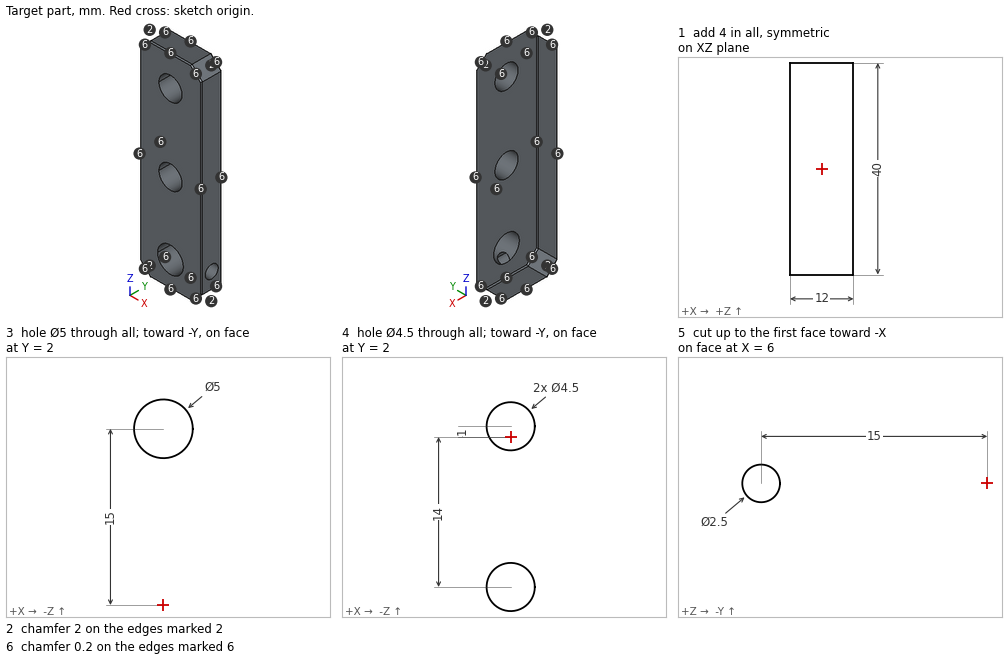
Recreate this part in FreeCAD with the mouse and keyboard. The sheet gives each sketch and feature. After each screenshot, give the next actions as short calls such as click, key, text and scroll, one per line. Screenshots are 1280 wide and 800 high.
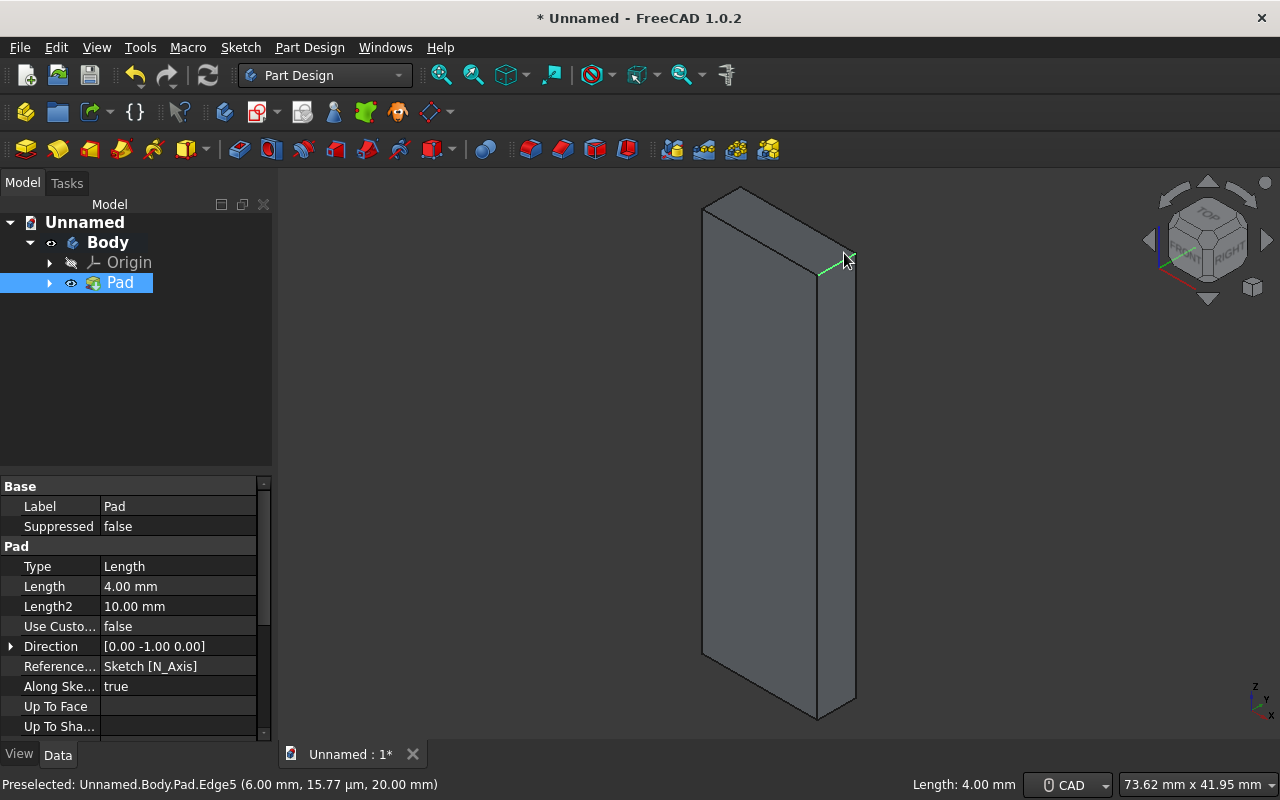
key(2)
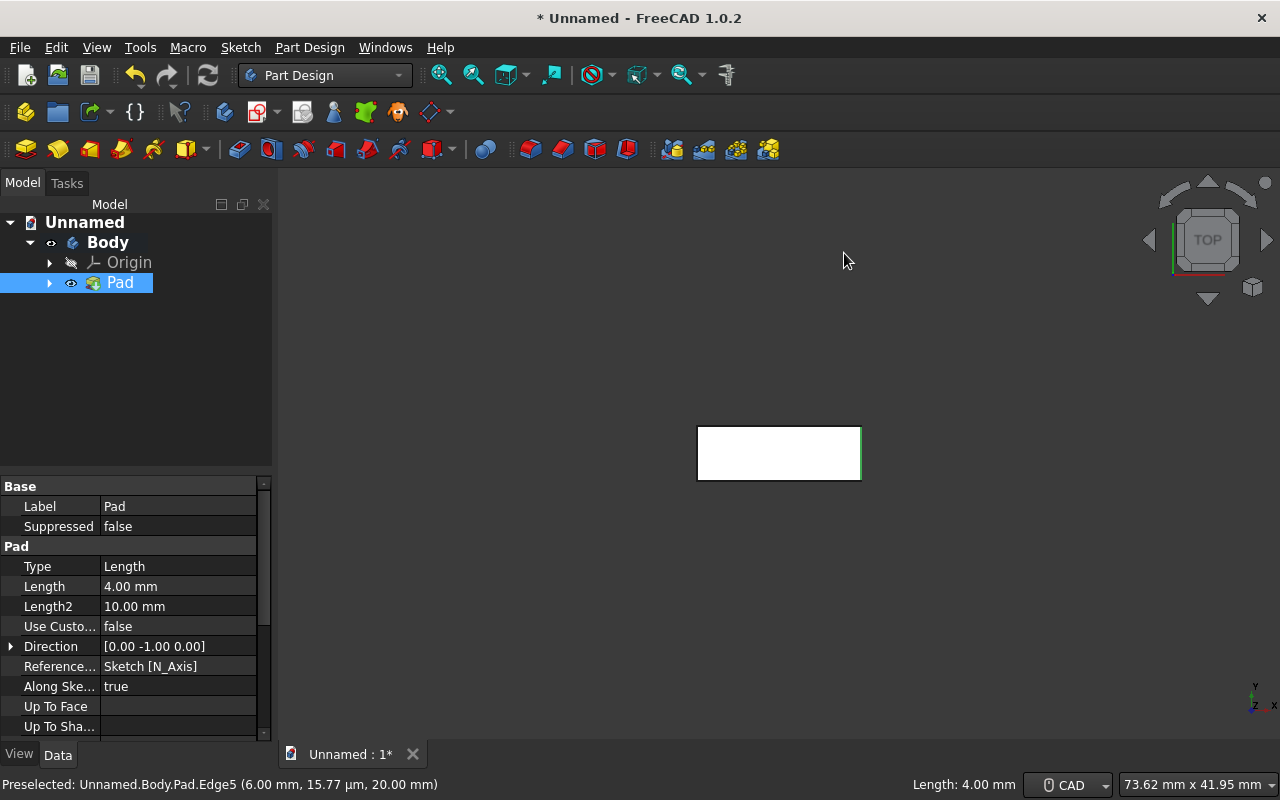
click(442, 76)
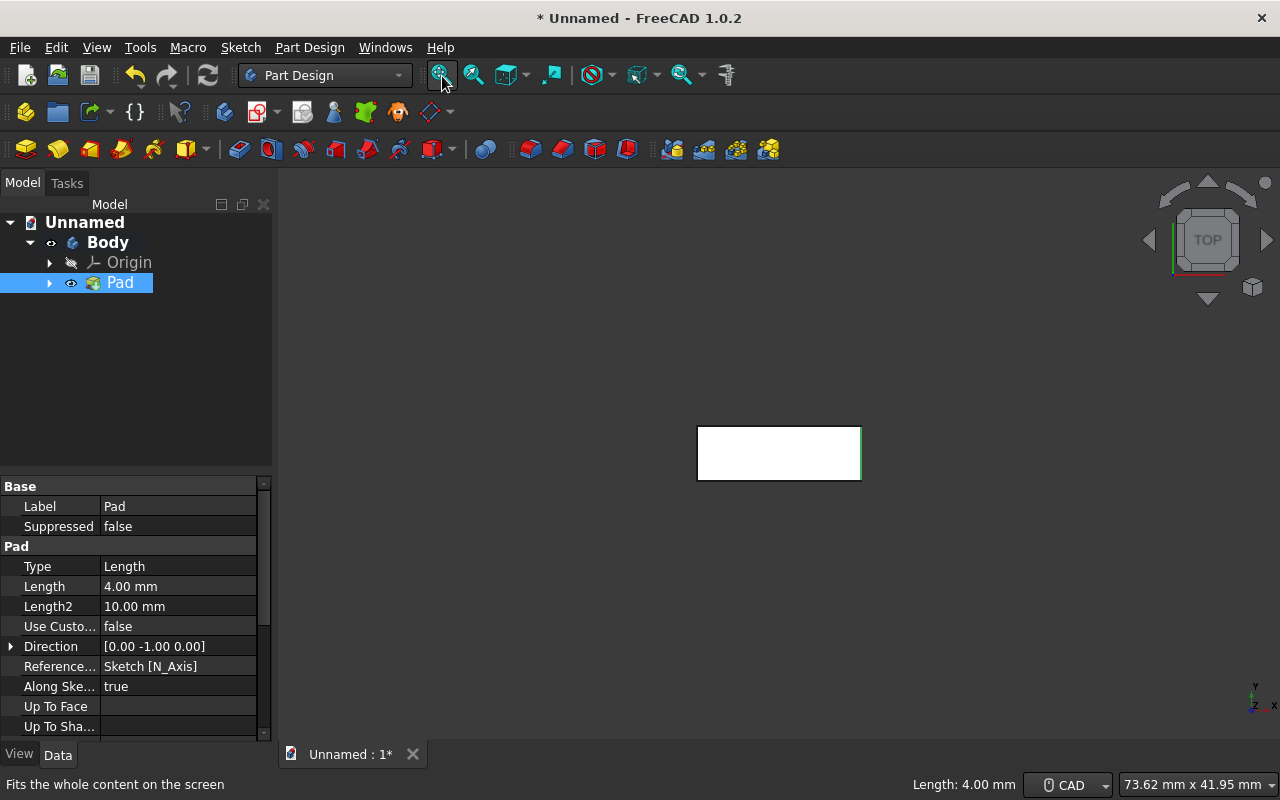
click(697, 452, ctrl)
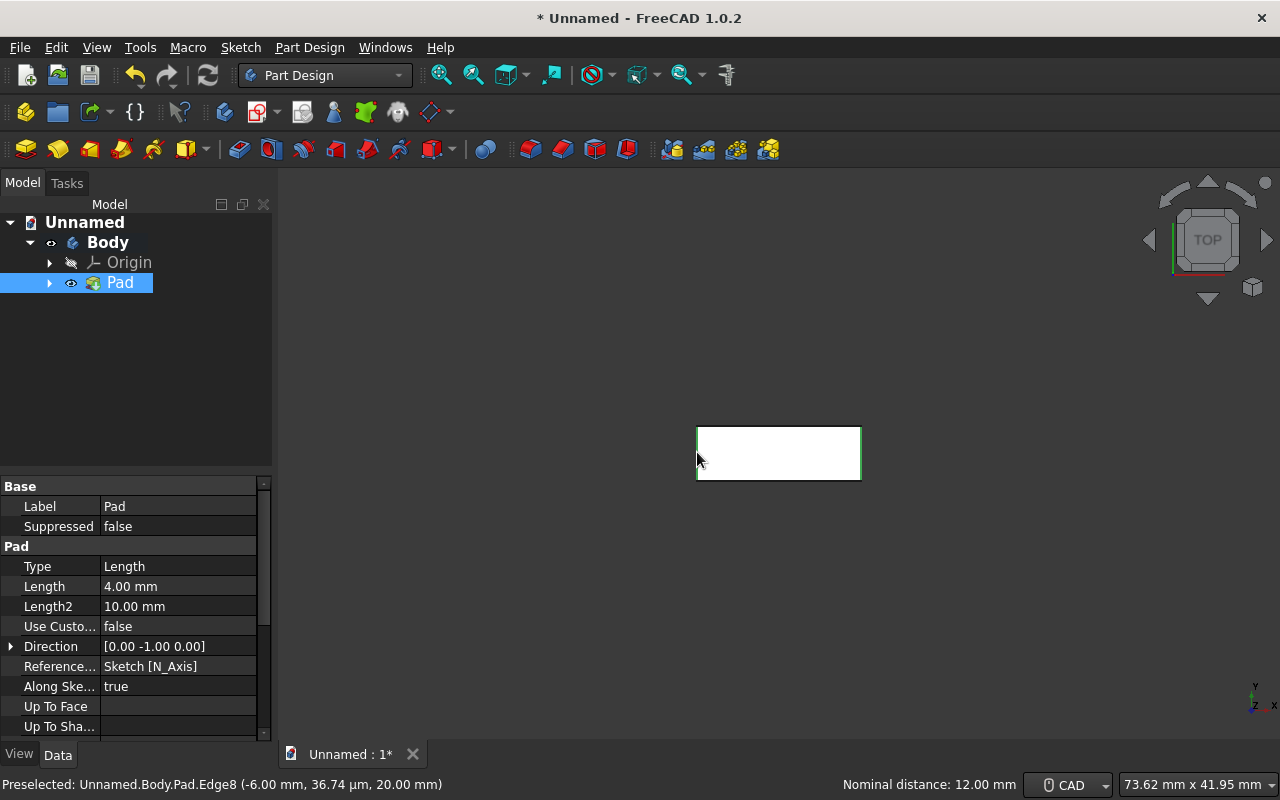
key(1)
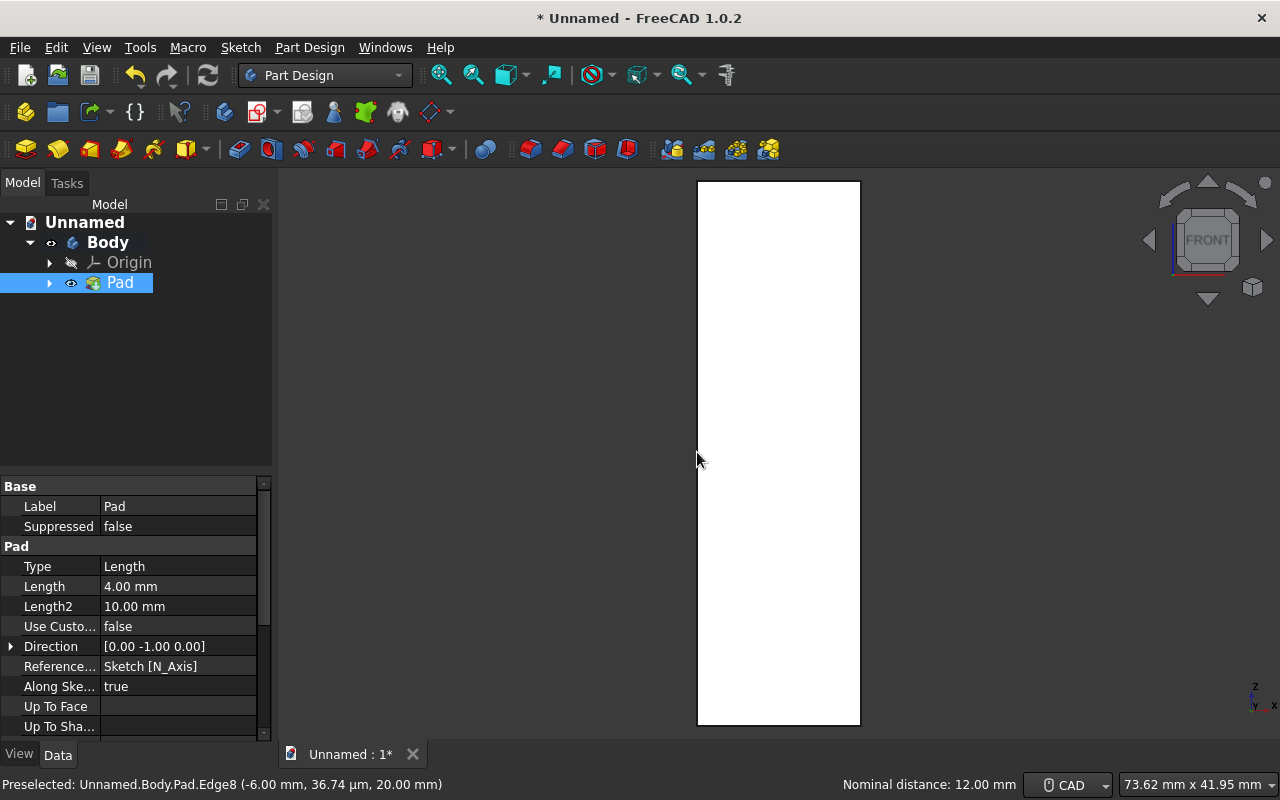
key(3)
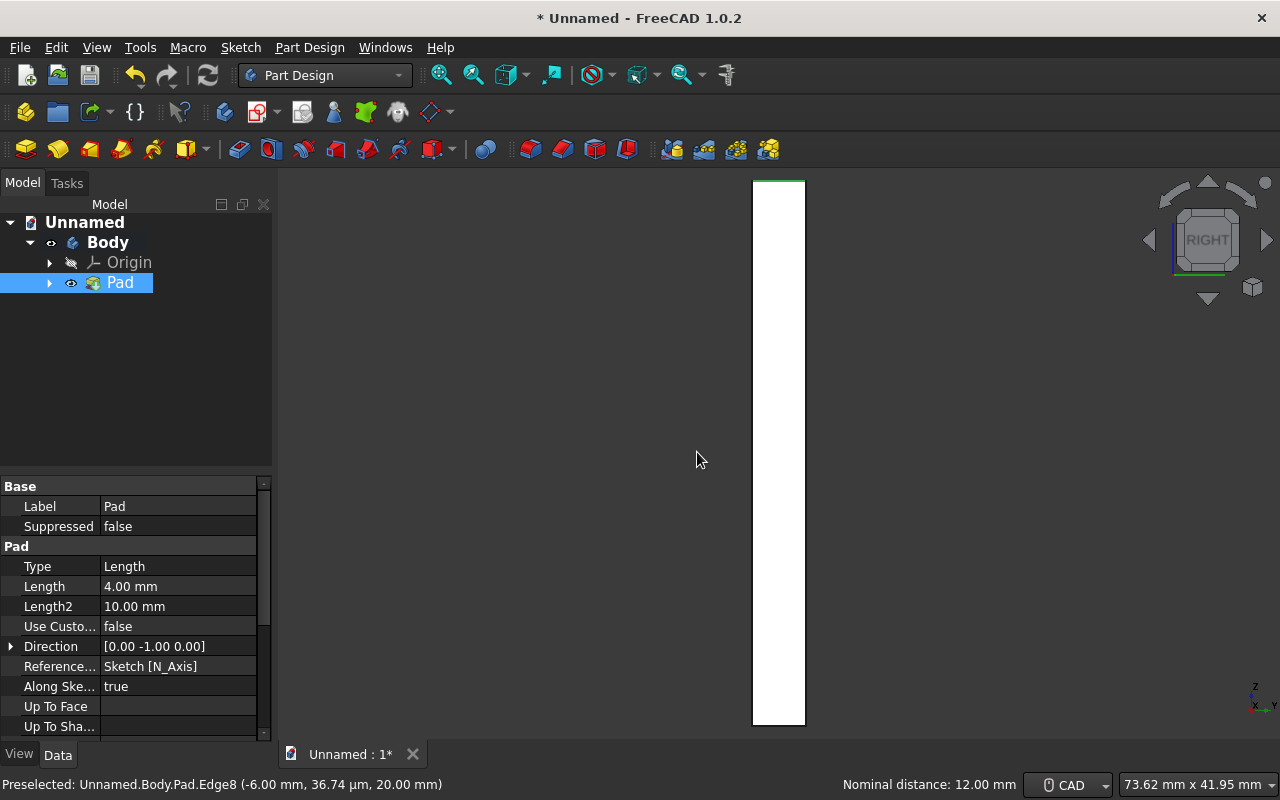
key(5)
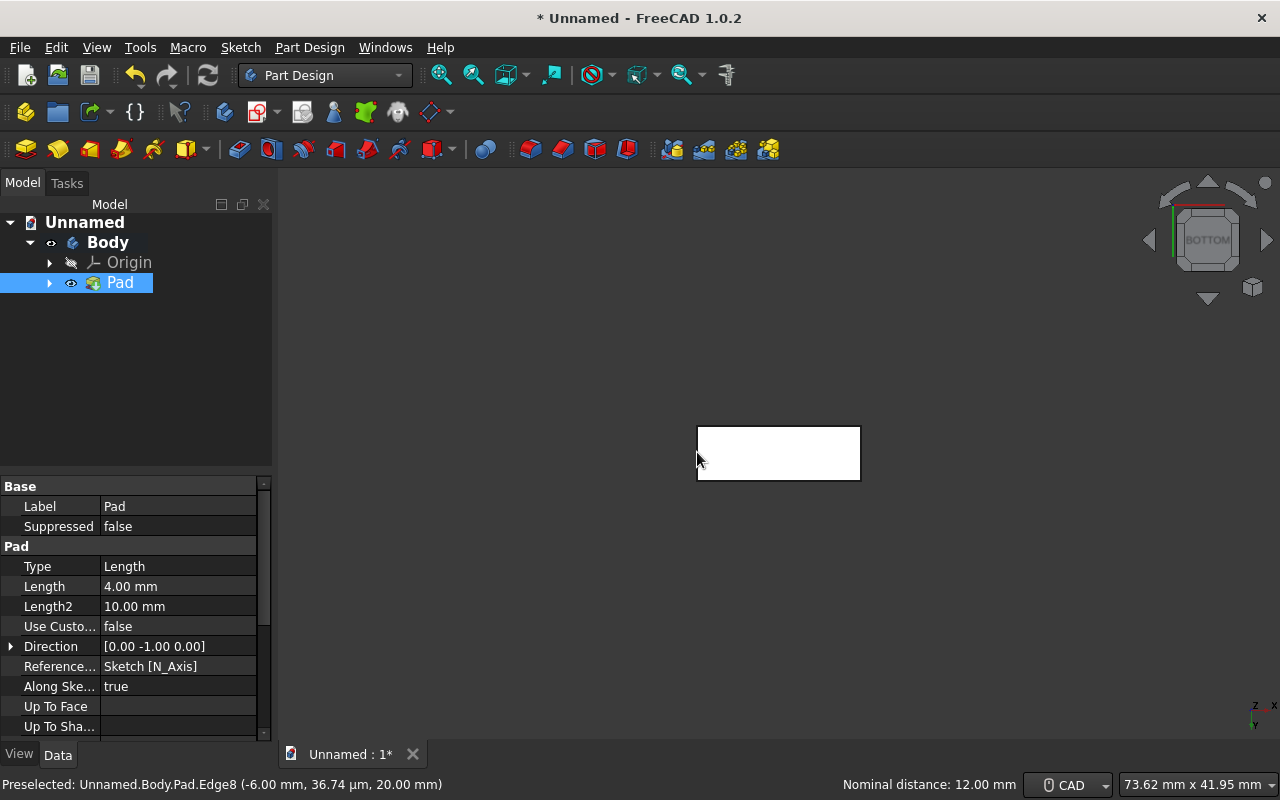
click(442, 76)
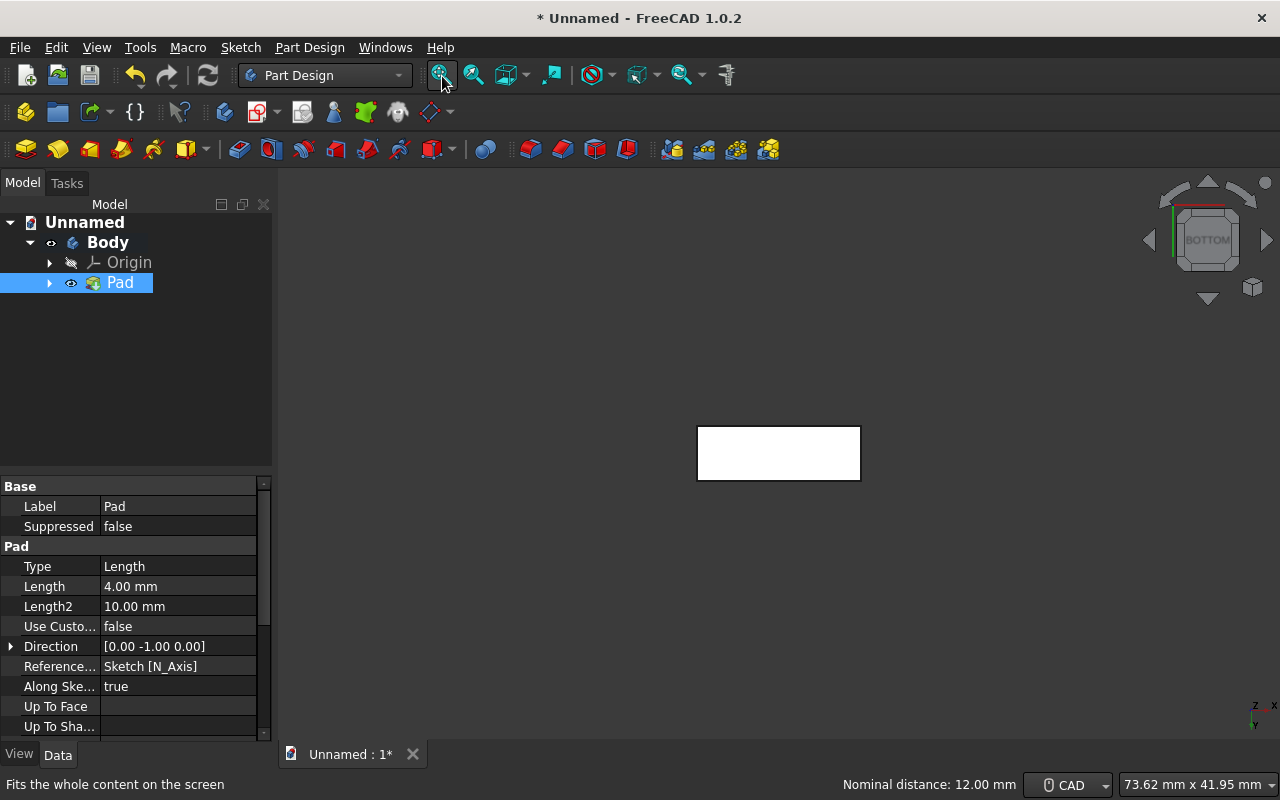
click(697, 452, ctrl)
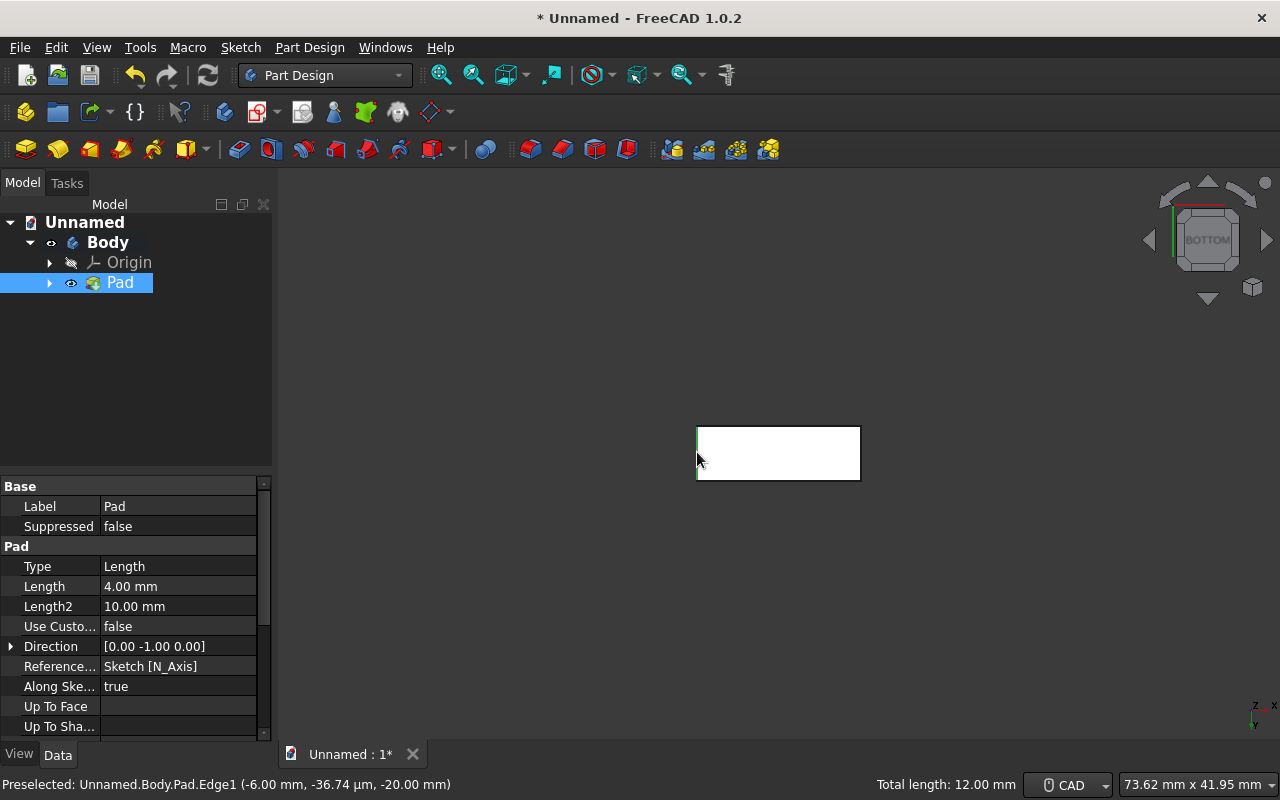
click(861, 452, ctrl)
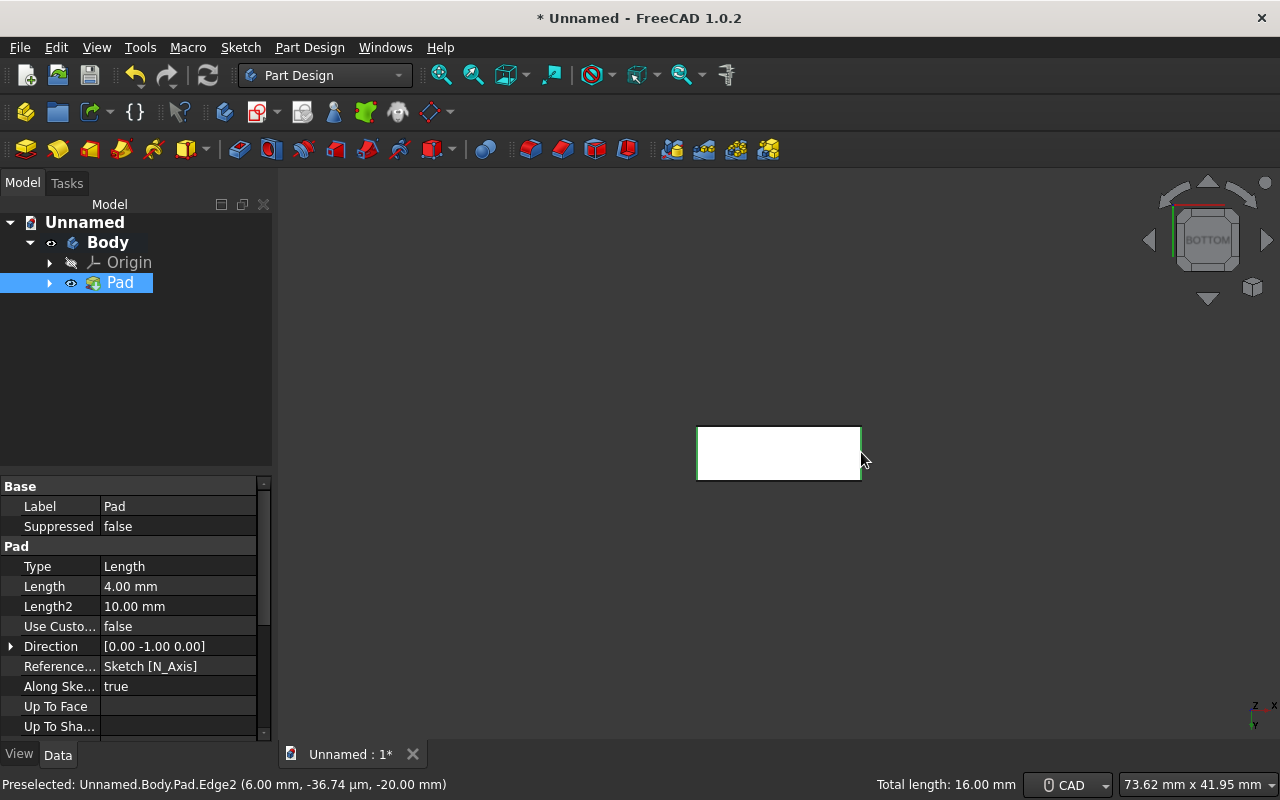
click(564, 150)